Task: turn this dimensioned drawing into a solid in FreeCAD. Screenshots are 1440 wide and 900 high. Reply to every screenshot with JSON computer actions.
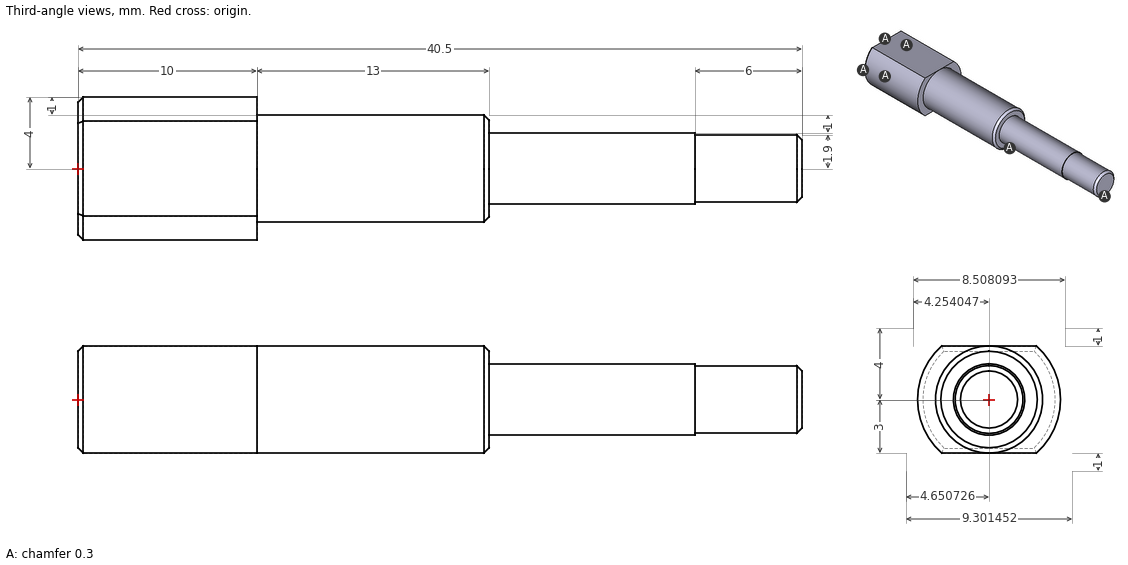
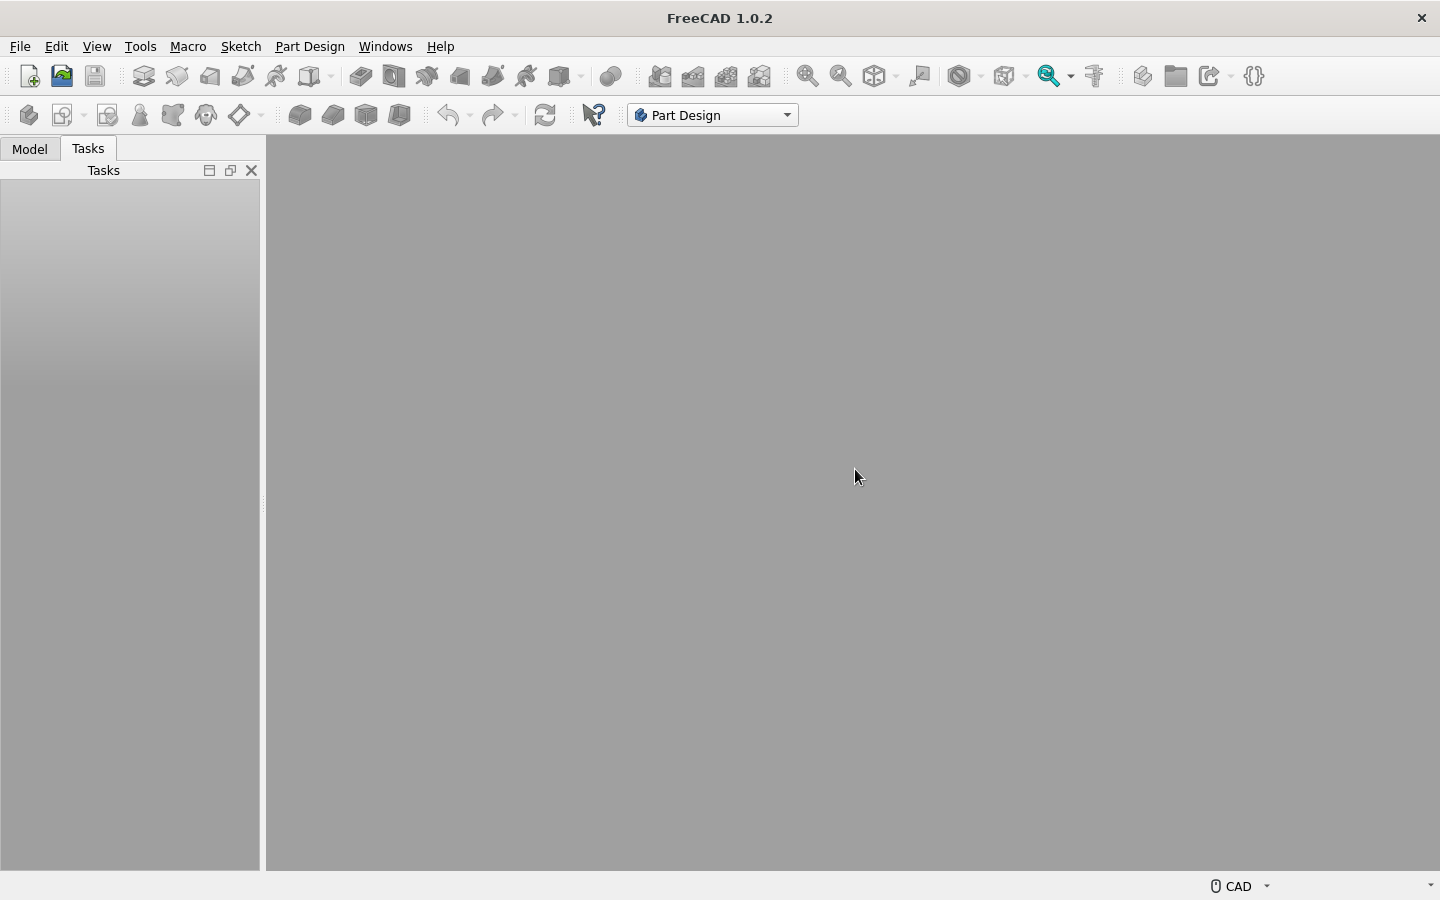
{"action": "key", "text": "ctrl+n"}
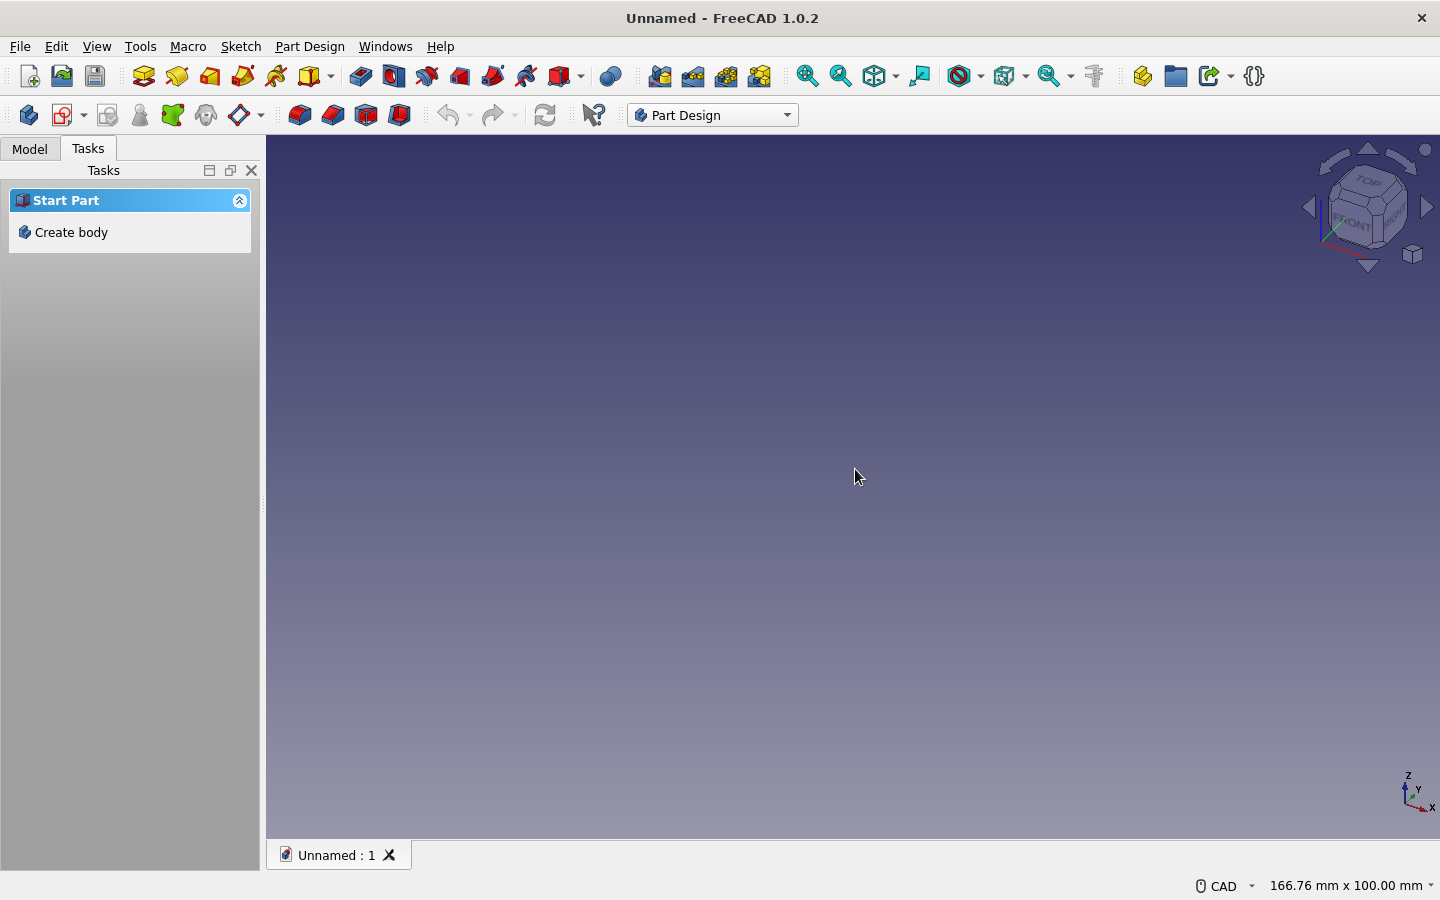
{"action": "left_click", "coordinate": [62, 116]}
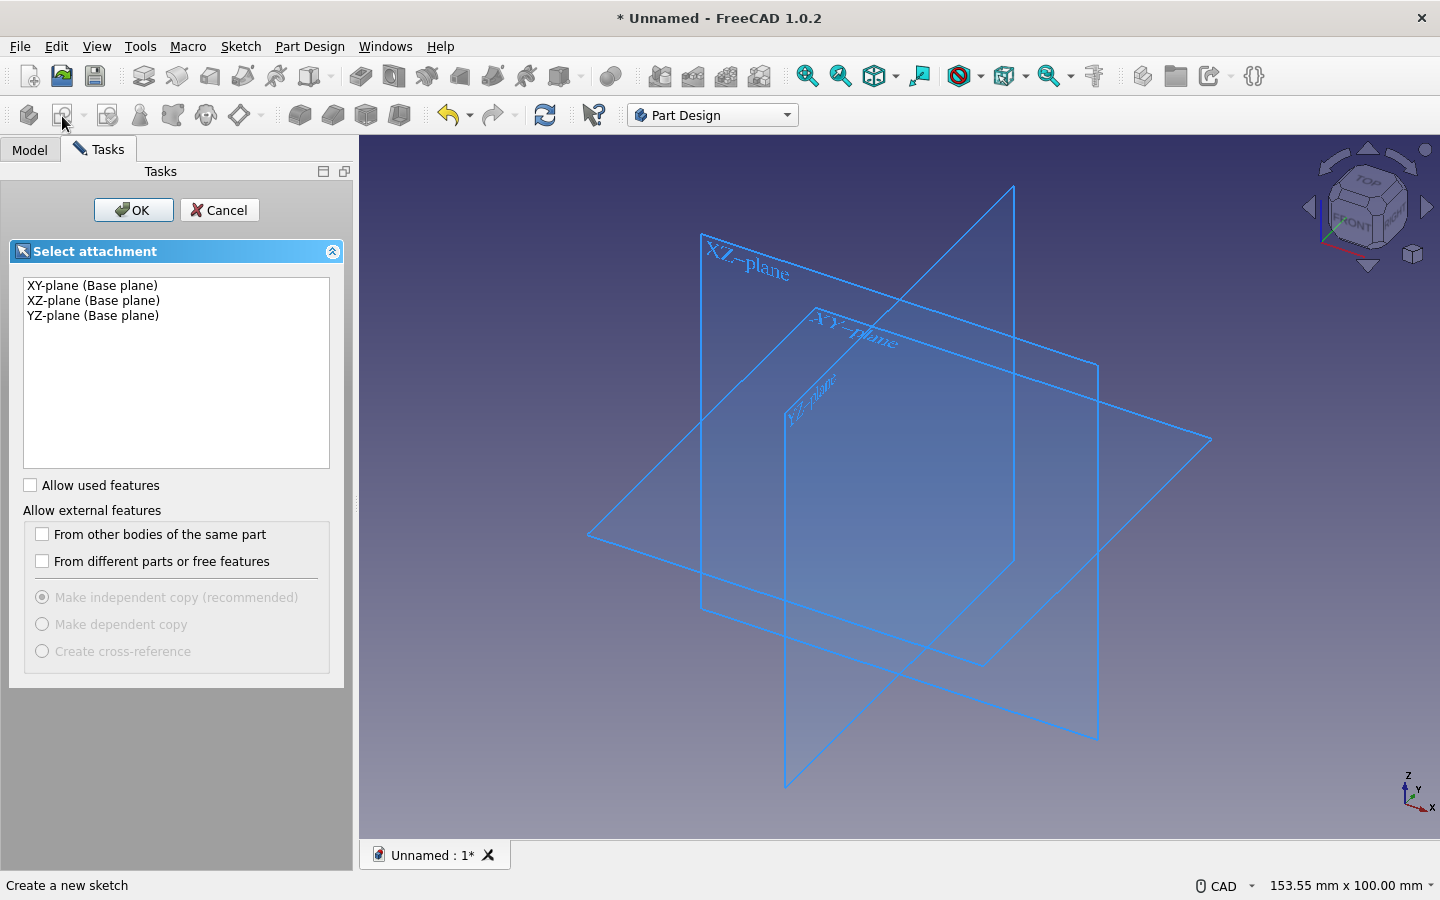
{"action": "left_click", "coordinate": [84, 286]}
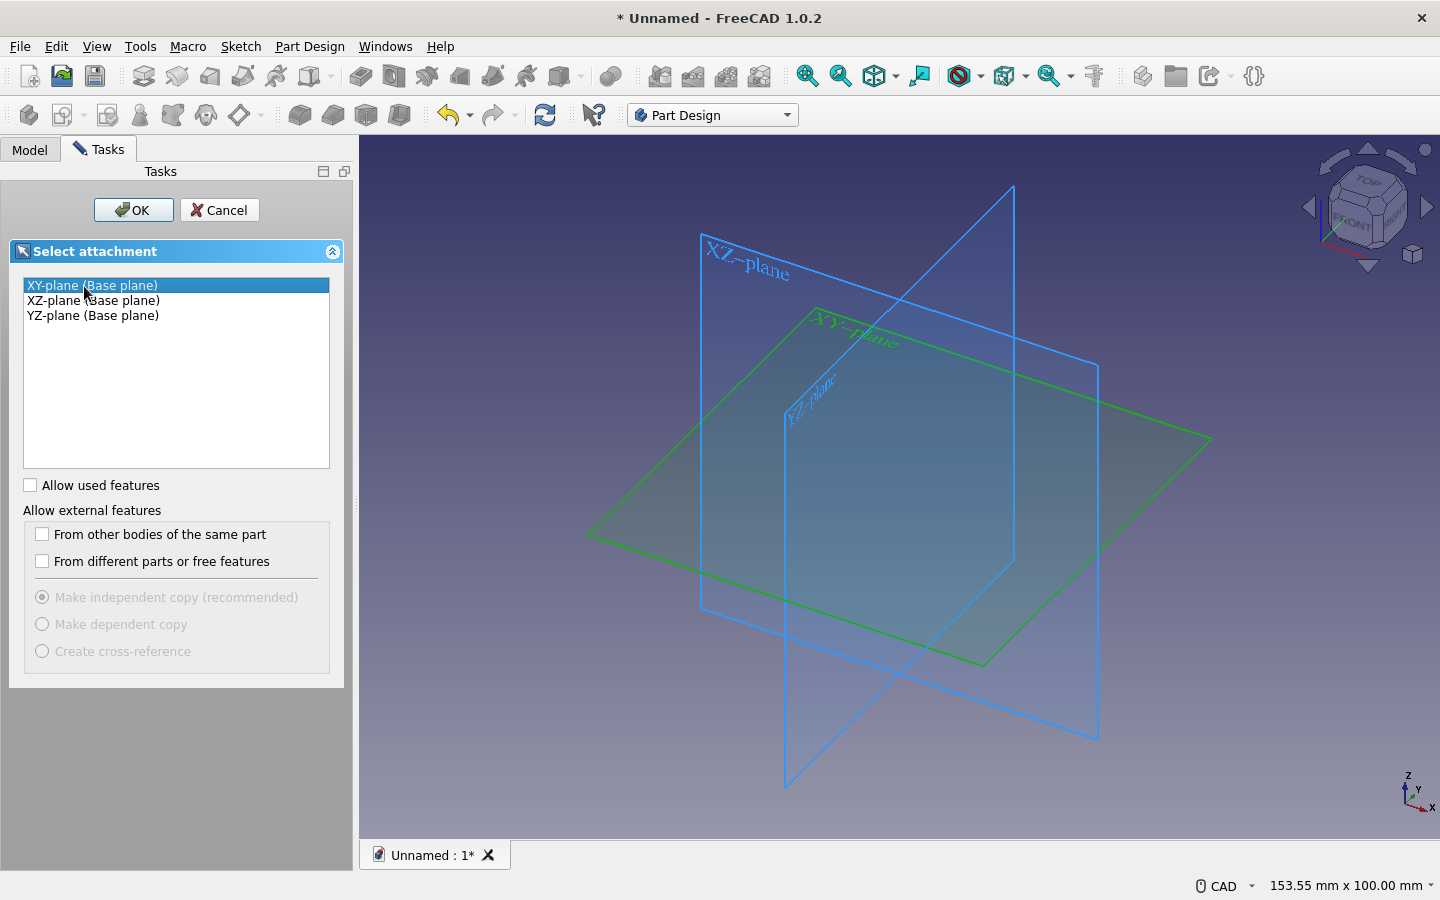
{"action": "left_click", "coordinate": [134, 210]}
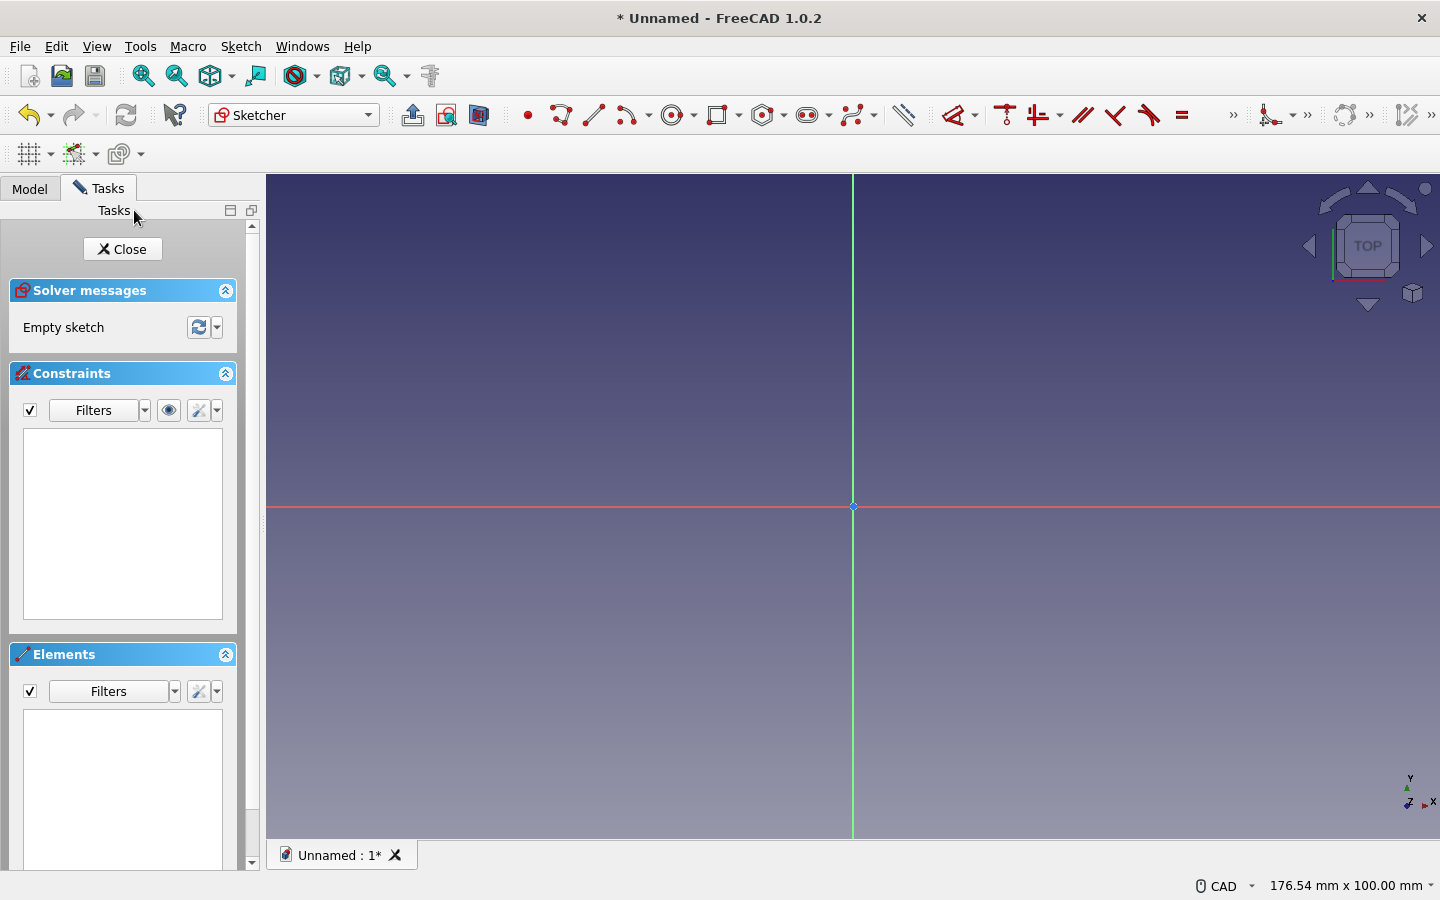
{"action": "scroll", "coordinate": [1106, 485], "scroll_direction": "up", "scroll_amount": 5}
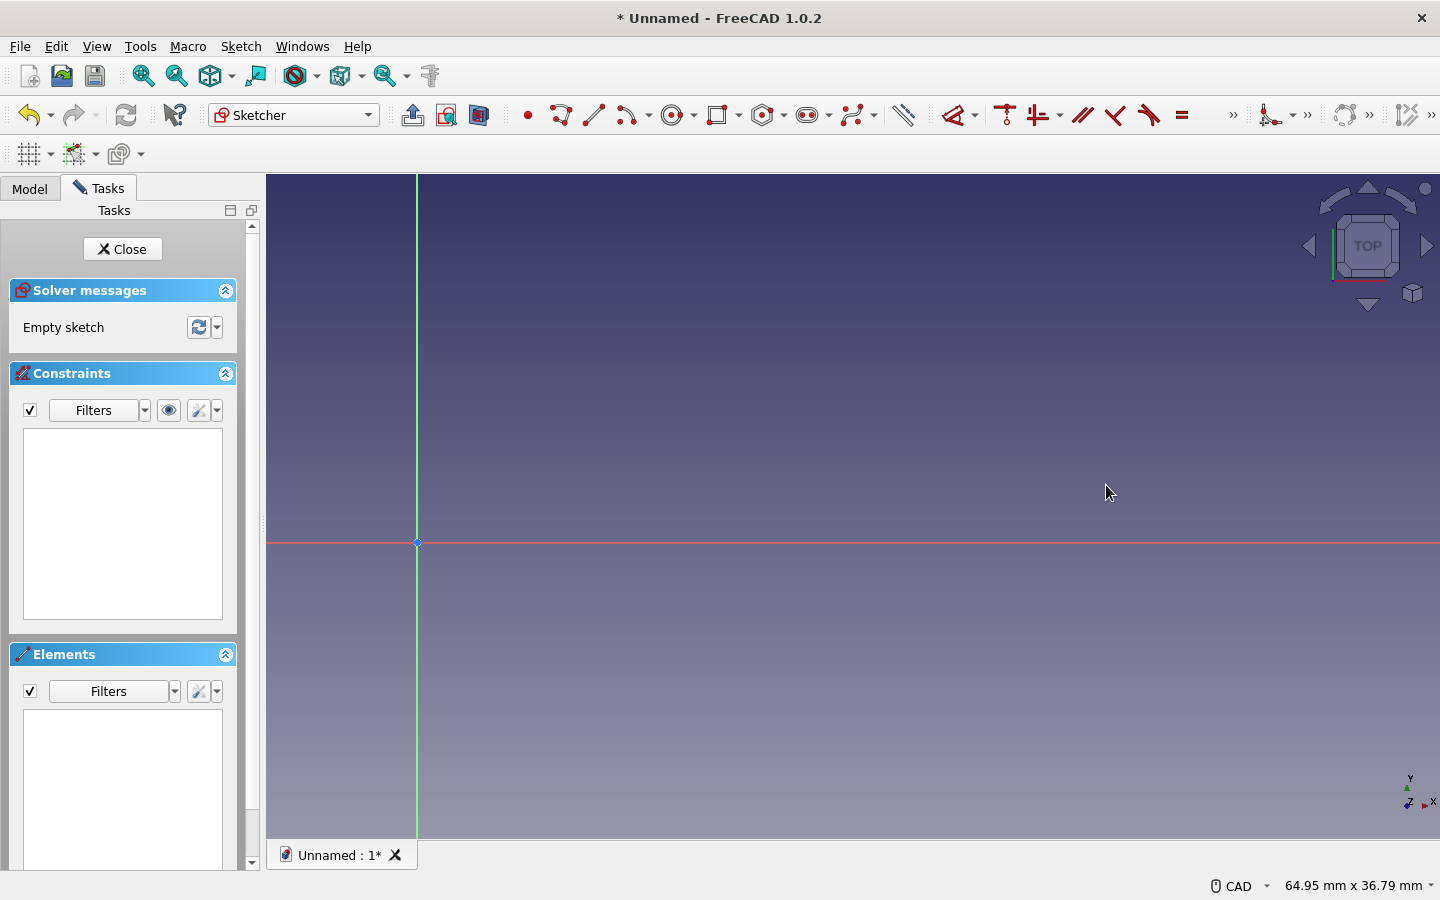
{"action": "key", "text": "g m"}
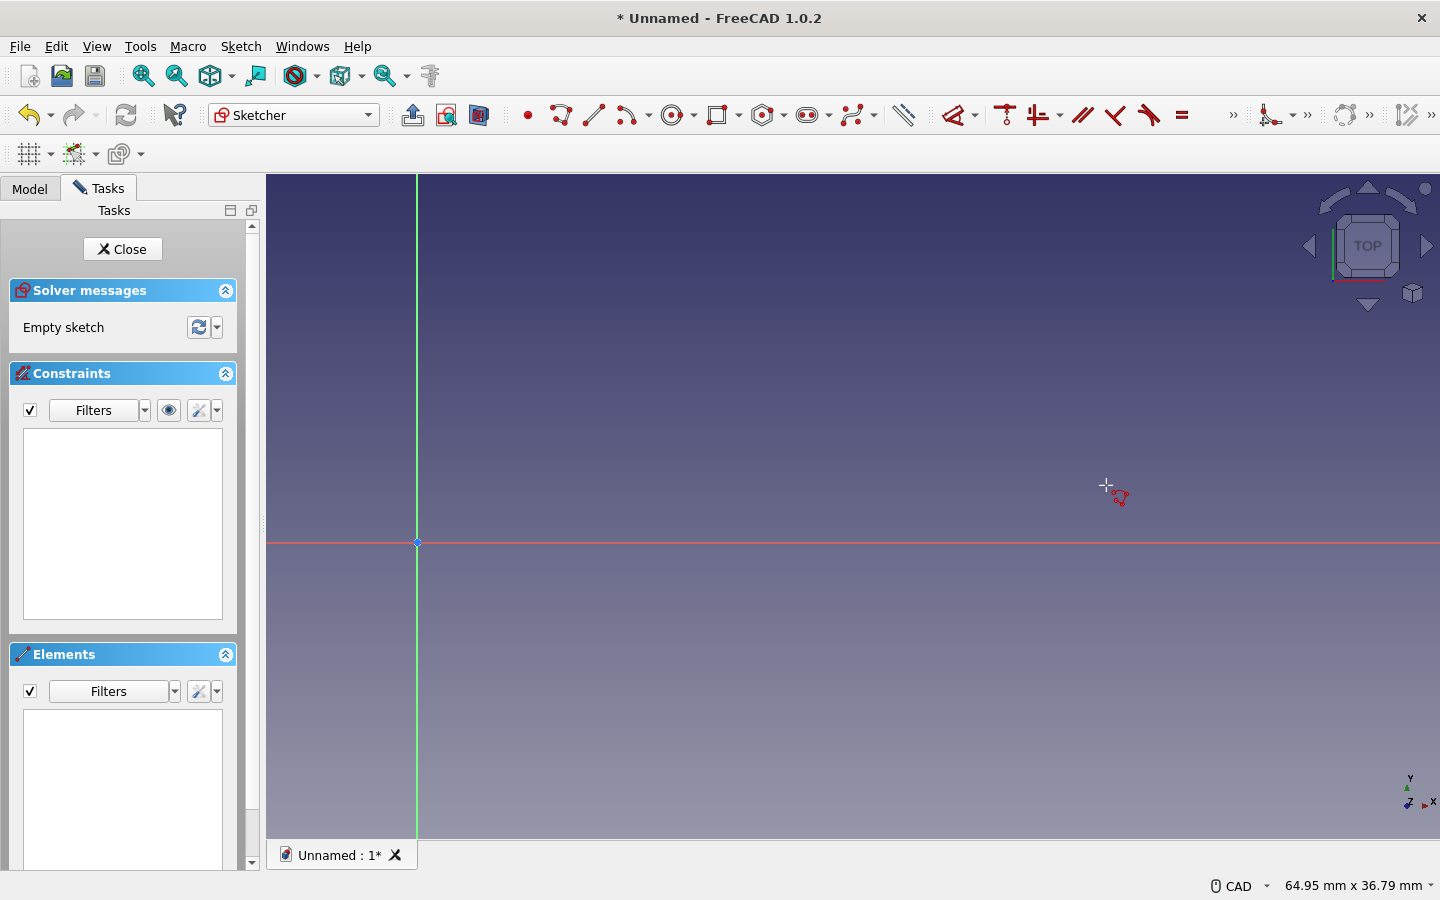
{"action": "left_click", "coordinate": [417, 543]}
{"action": "left_click", "coordinate": [1149, 534]}
{"action": "left_click", "coordinate": [1149, 508]}
{"action": "left_click", "coordinate": [1041, 508]}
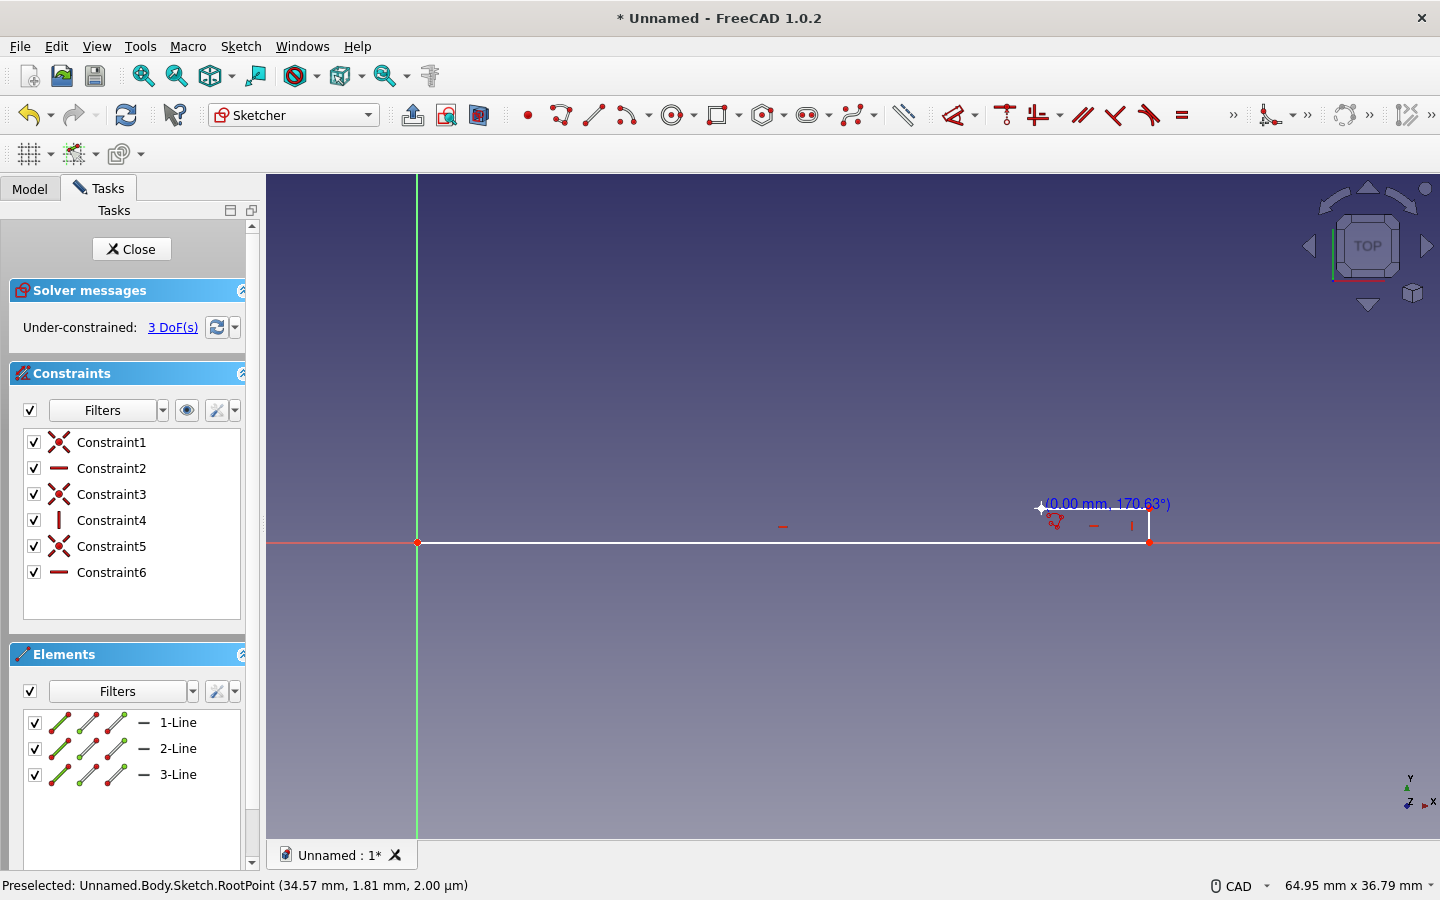
{"action": "scroll", "coordinate": [1041, 506], "scroll_direction": "up", "scroll_amount": 11}